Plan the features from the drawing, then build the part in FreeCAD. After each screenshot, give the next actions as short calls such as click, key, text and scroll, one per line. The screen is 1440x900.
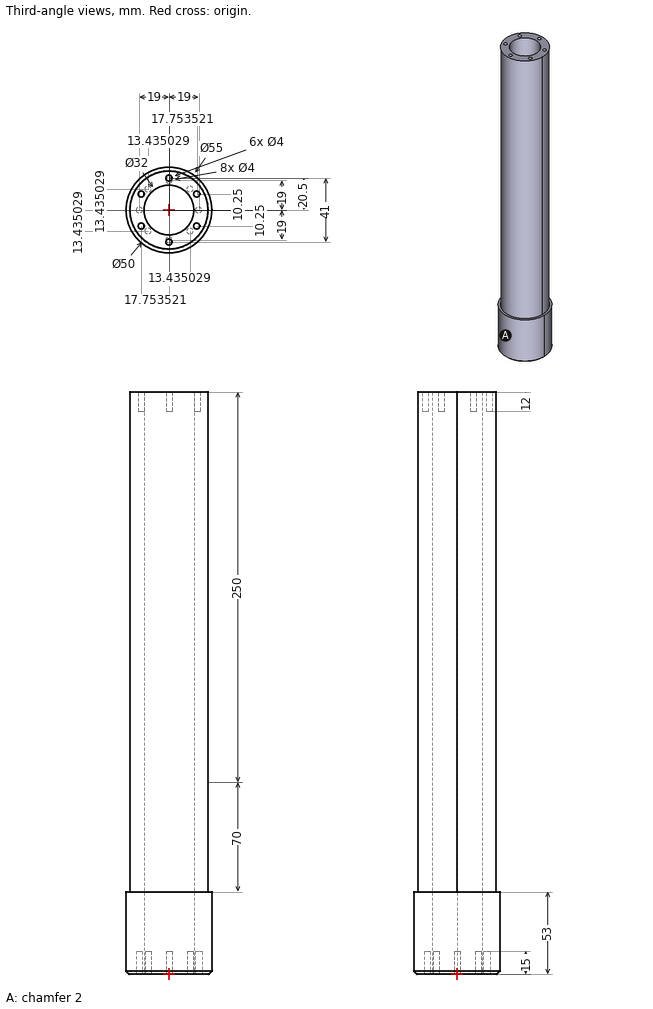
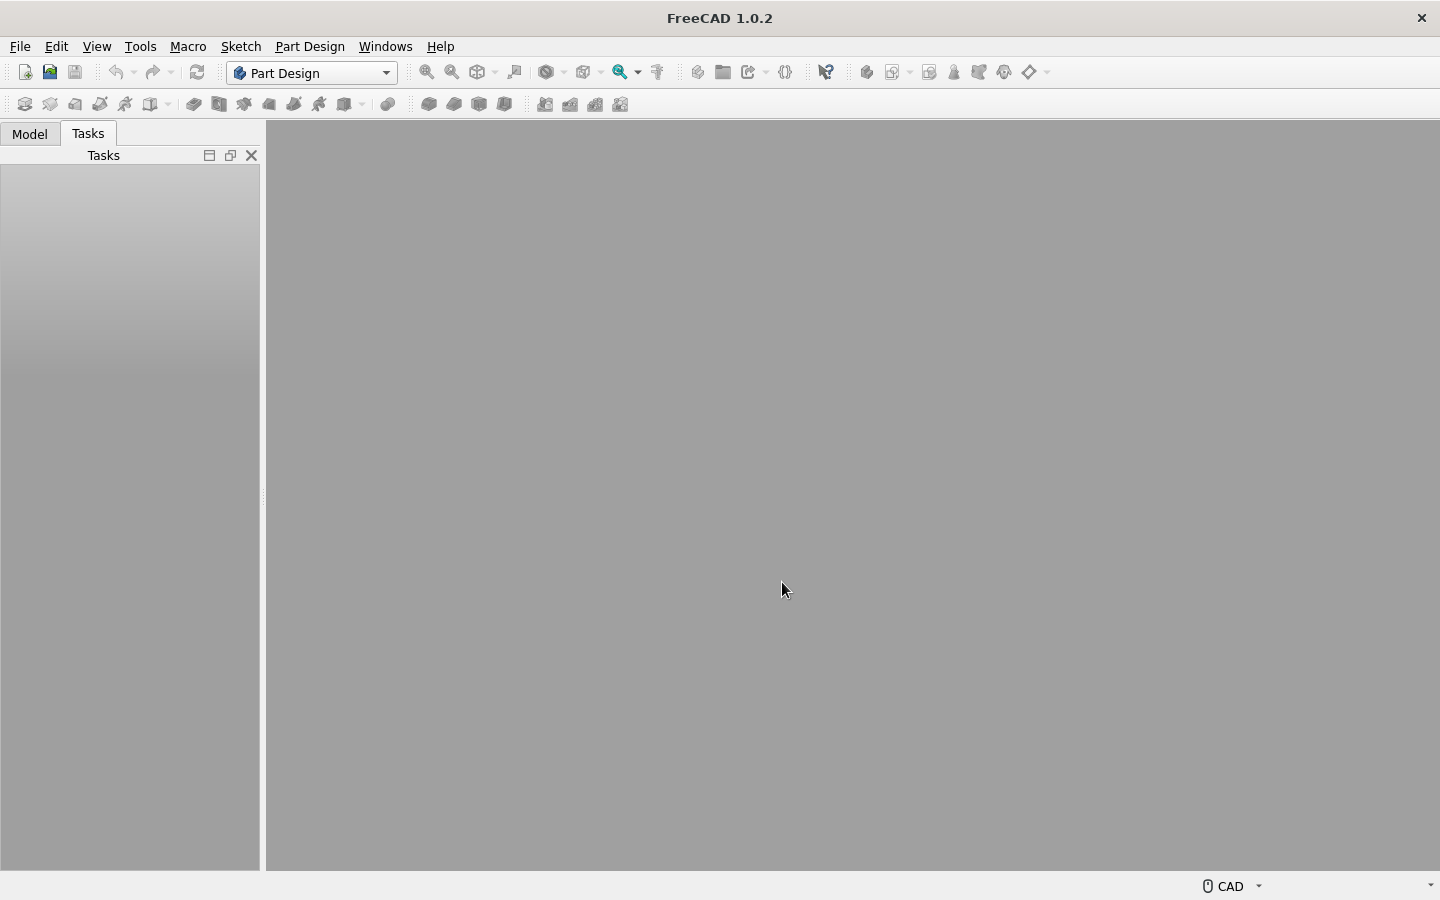
click(25, 72)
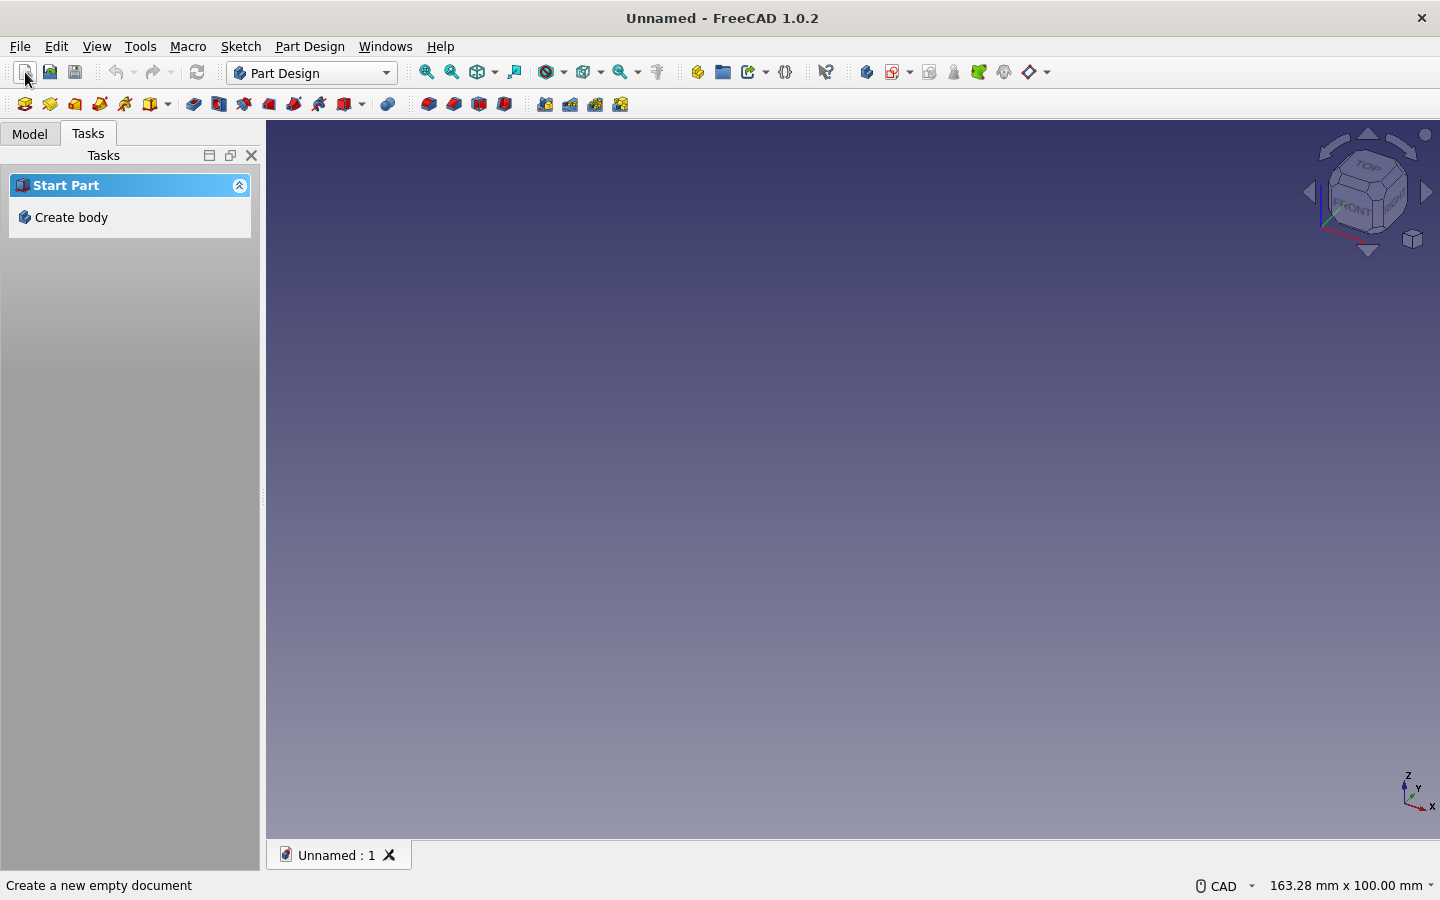
click(892, 72)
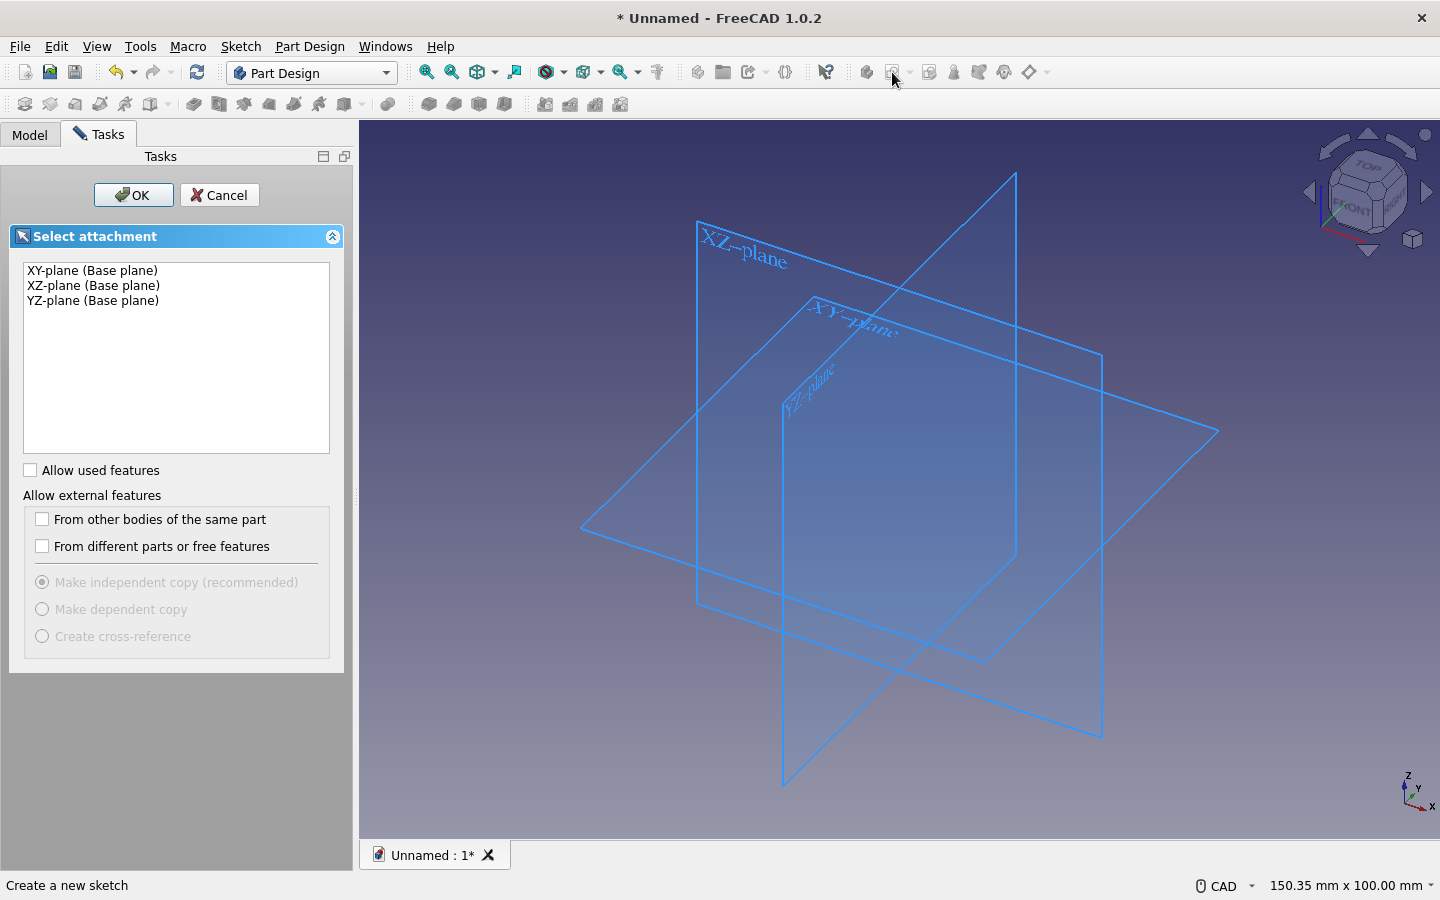
click(84, 270)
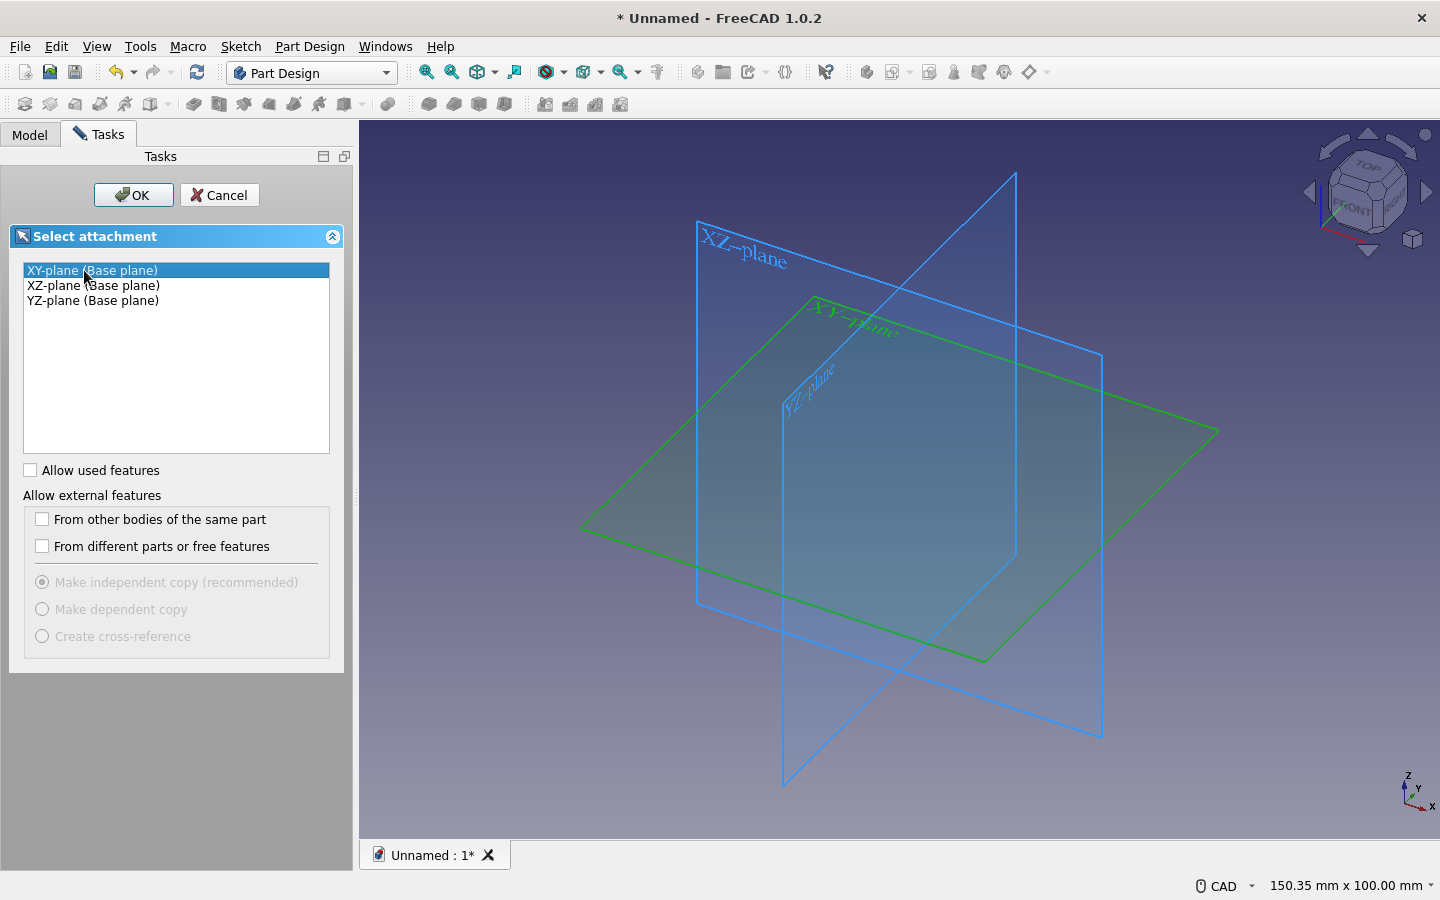
click(134, 195)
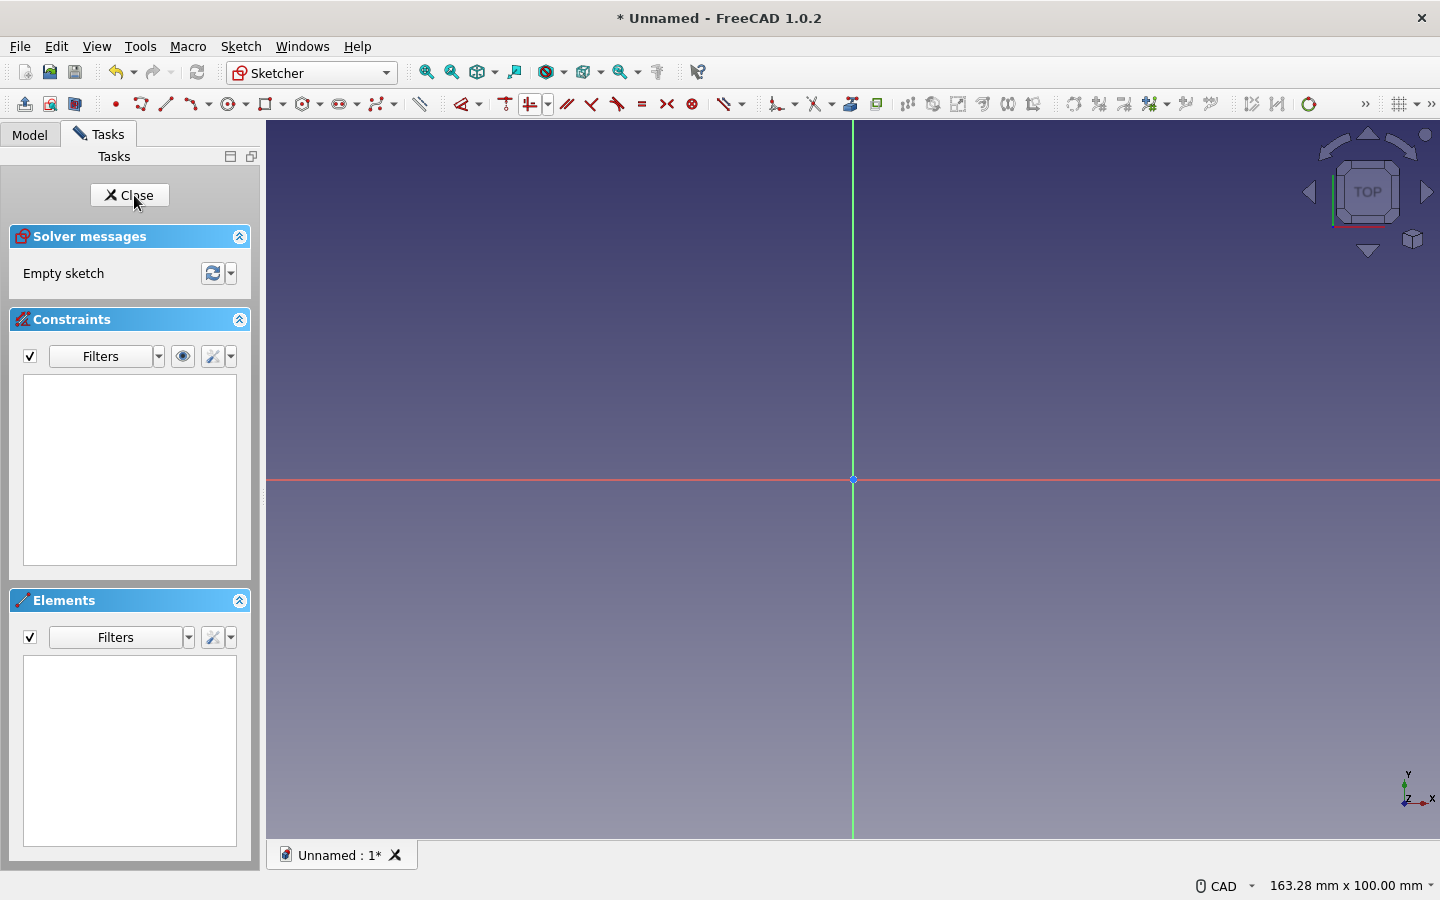
click(228, 104)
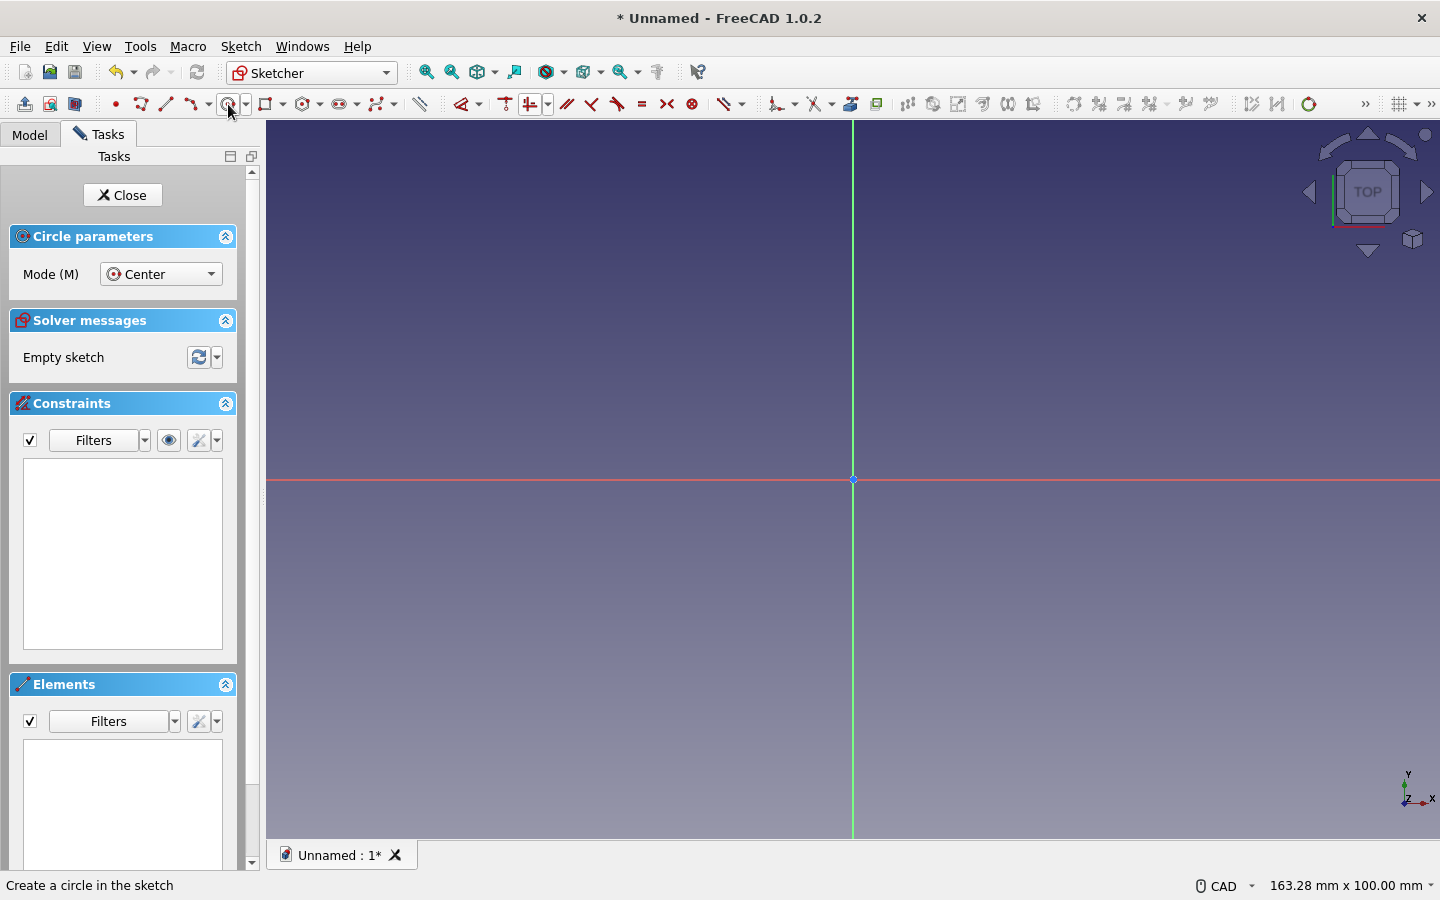
click(853, 480)
move(993, 340)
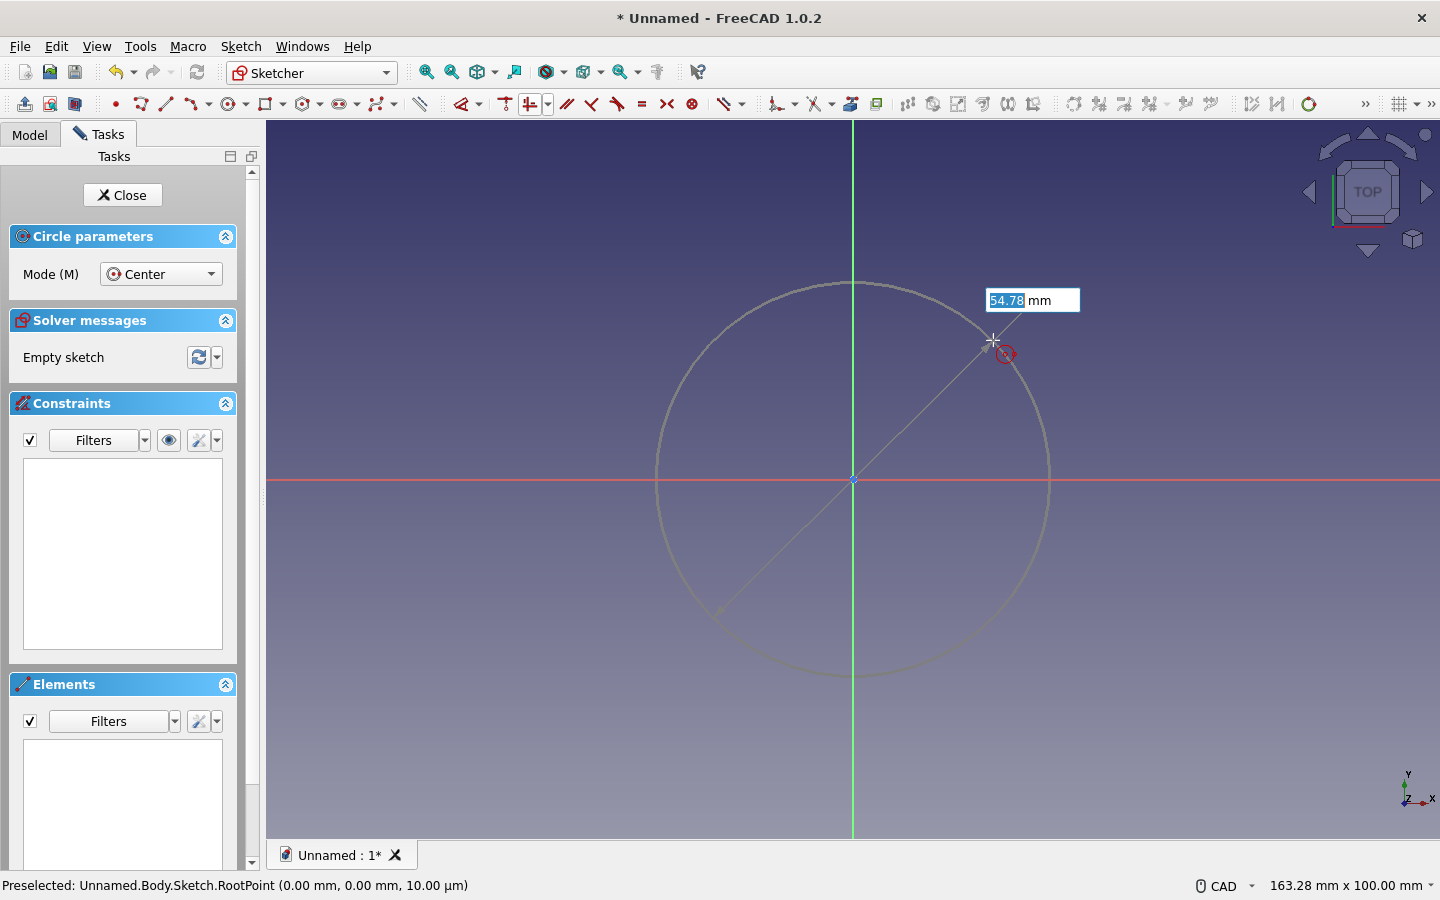
text(55)
key(Return)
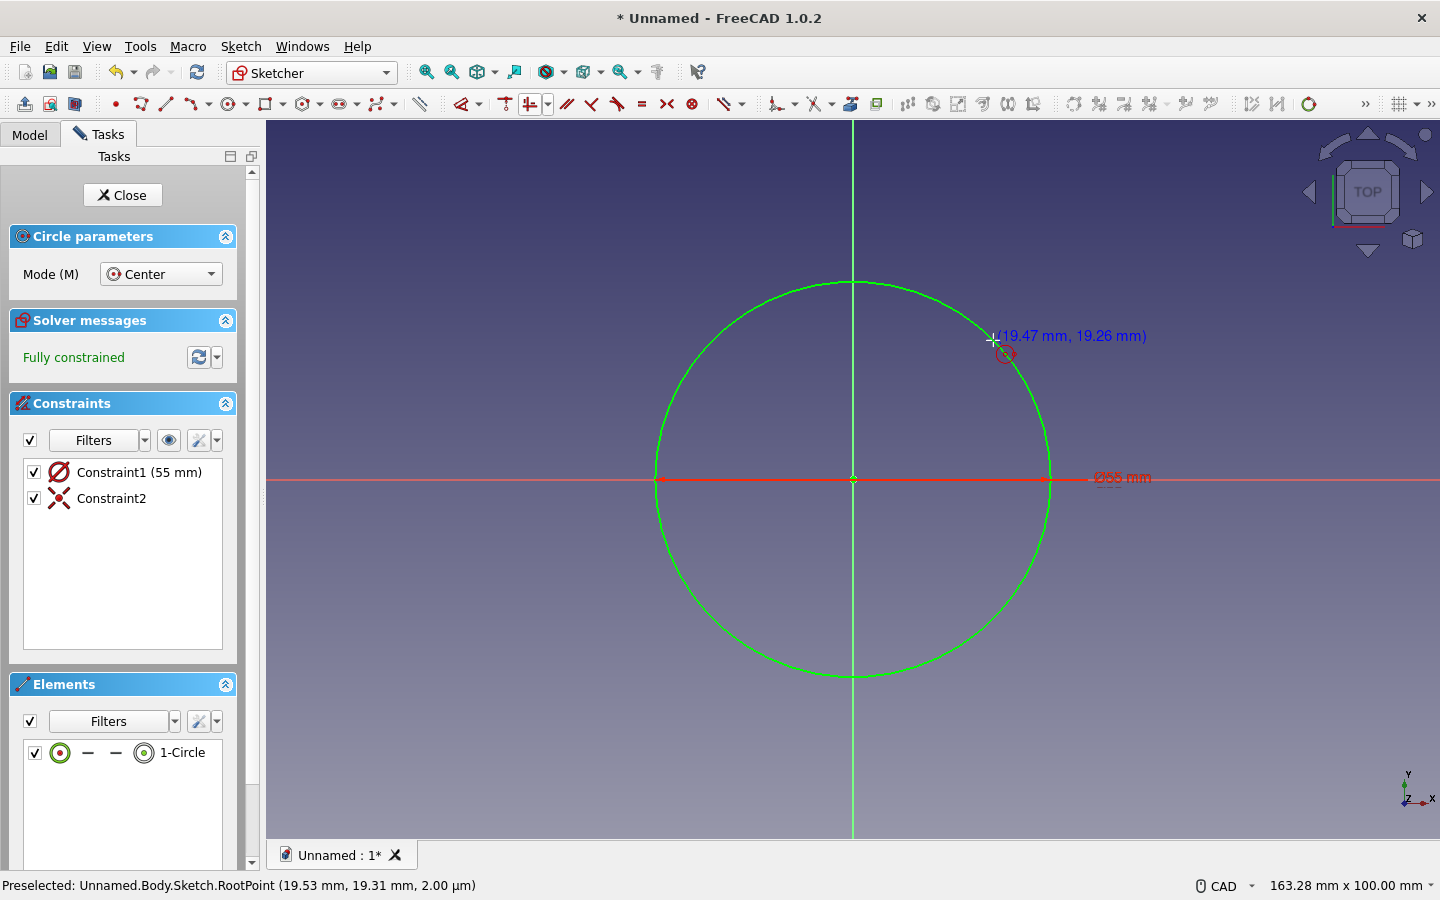
click(853, 480)
move(934, 398)